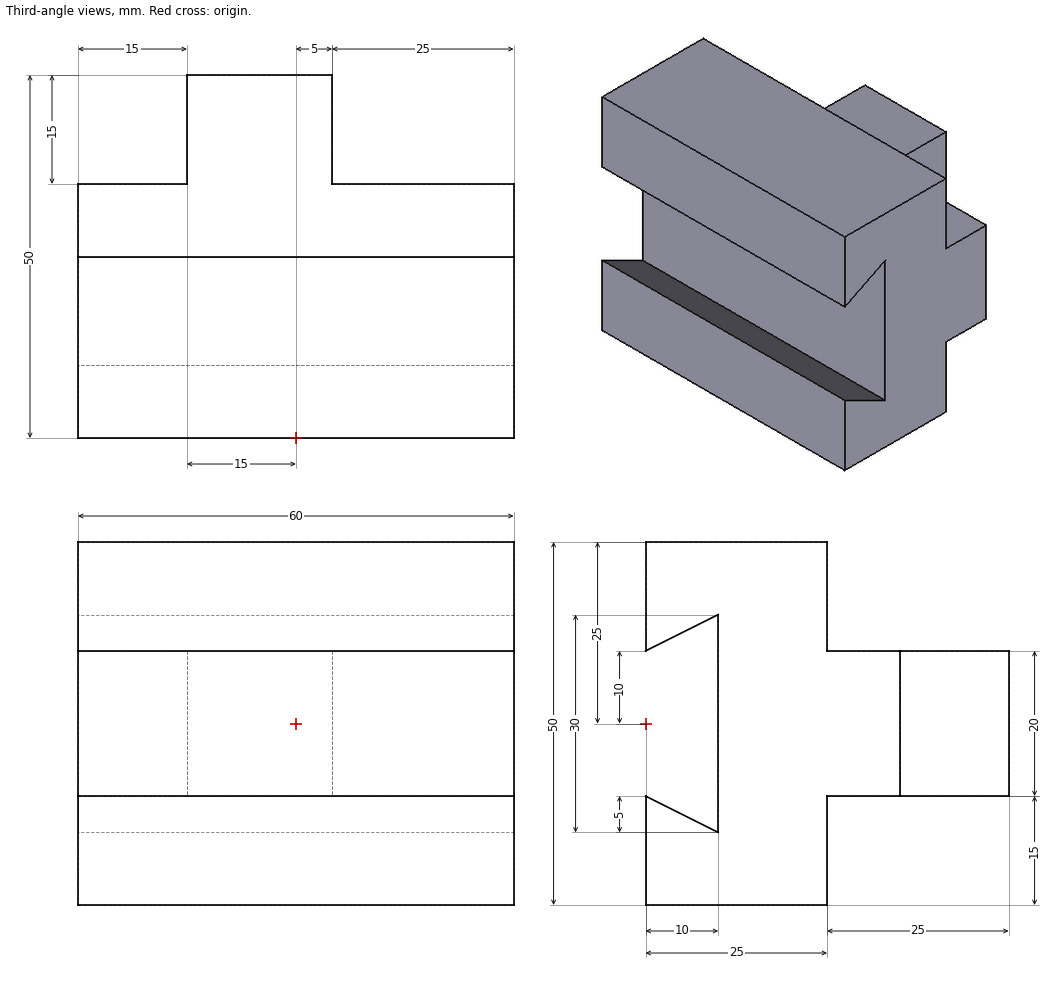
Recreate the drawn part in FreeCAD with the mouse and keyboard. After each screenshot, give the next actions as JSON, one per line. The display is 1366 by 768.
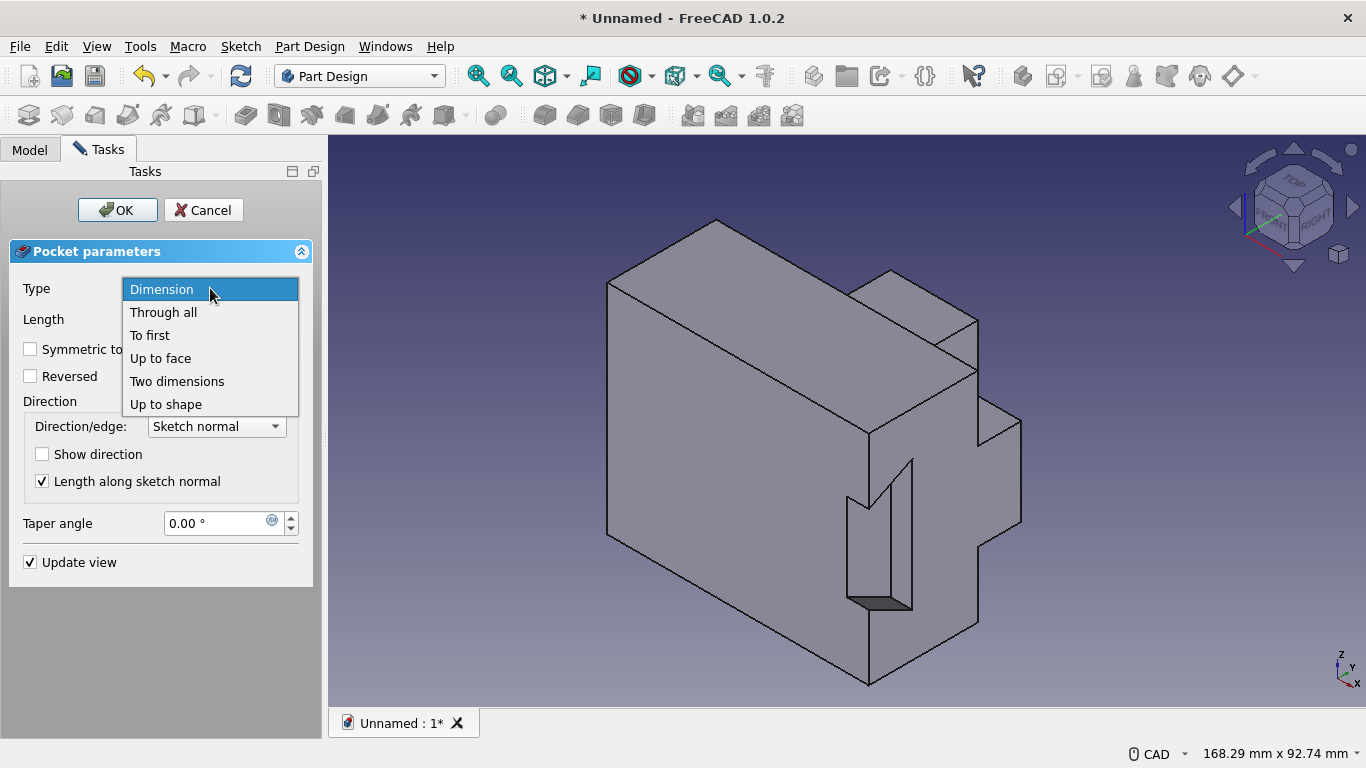
{"action": "left_click", "coordinate": [208, 336]}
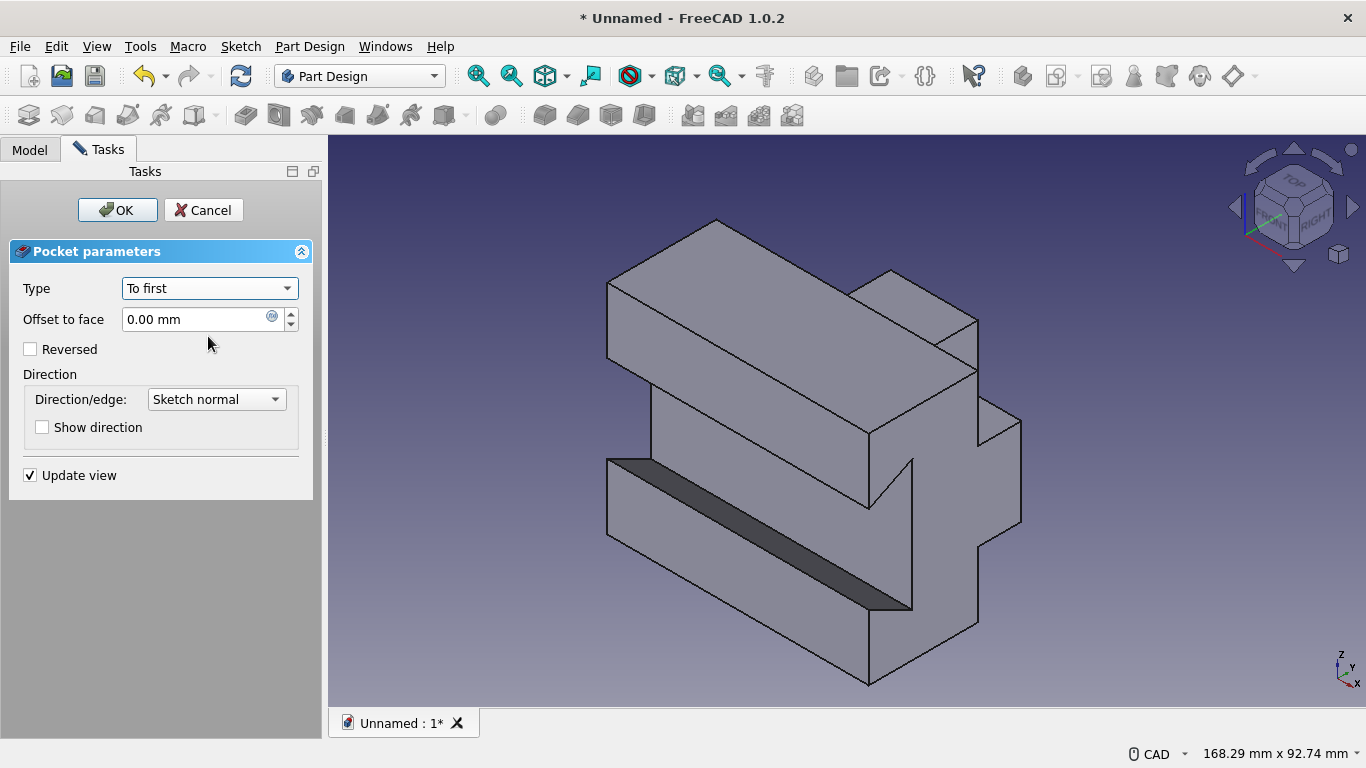
{"action": "left_click", "coordinate": [118, 210]}